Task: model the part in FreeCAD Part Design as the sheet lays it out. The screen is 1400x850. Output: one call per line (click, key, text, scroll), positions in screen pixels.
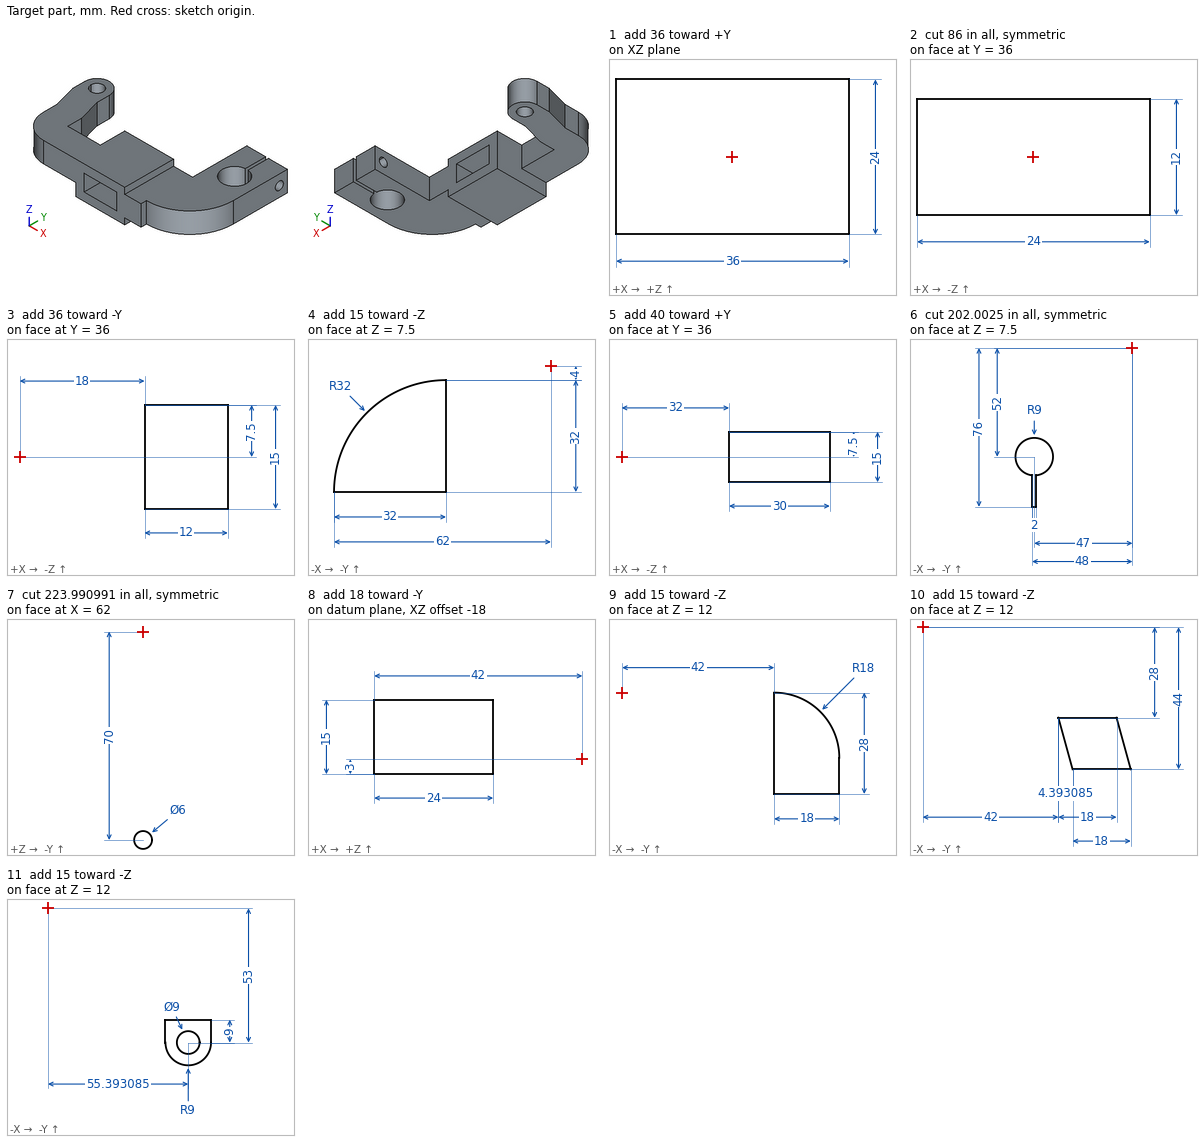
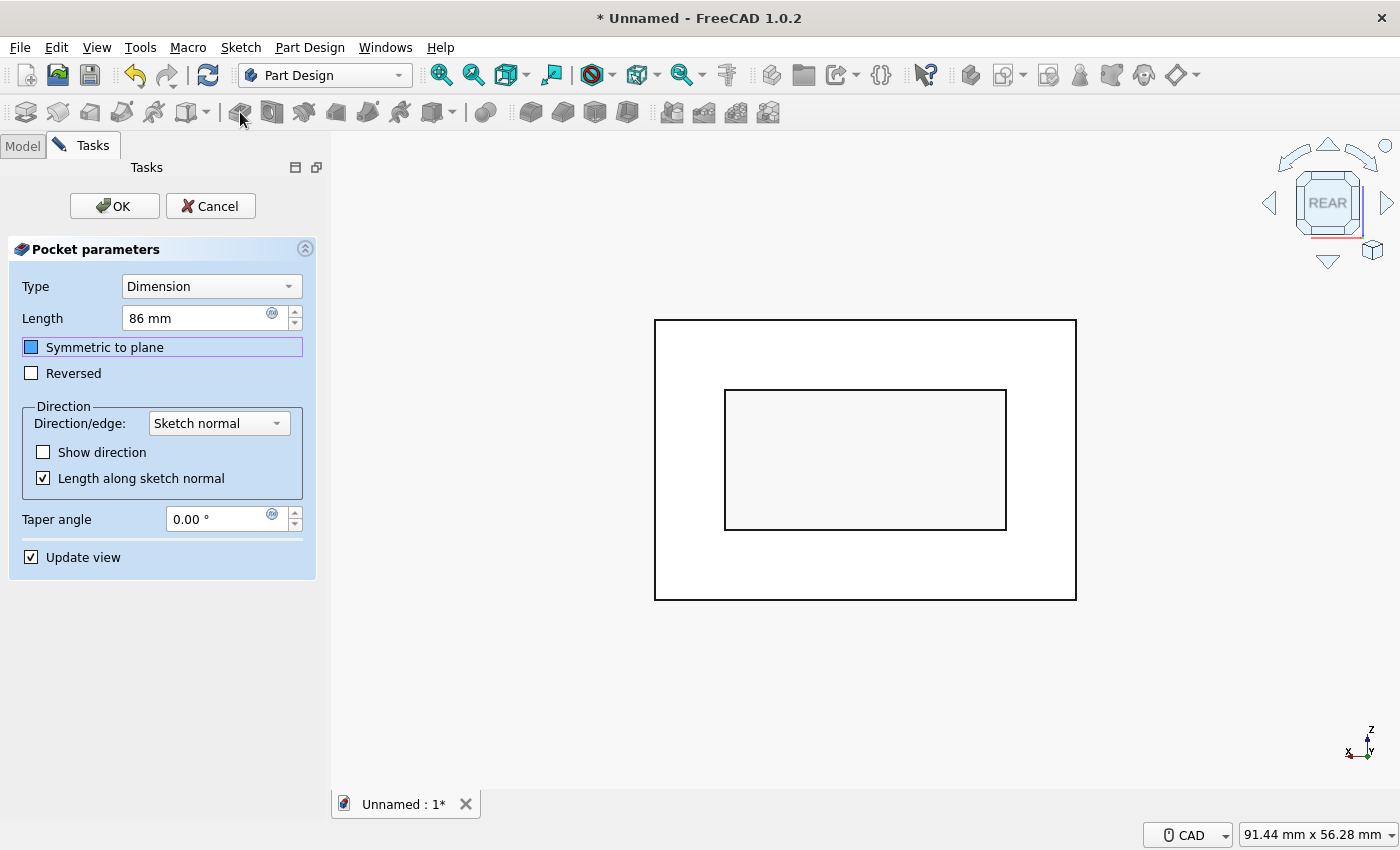
click(30, 347)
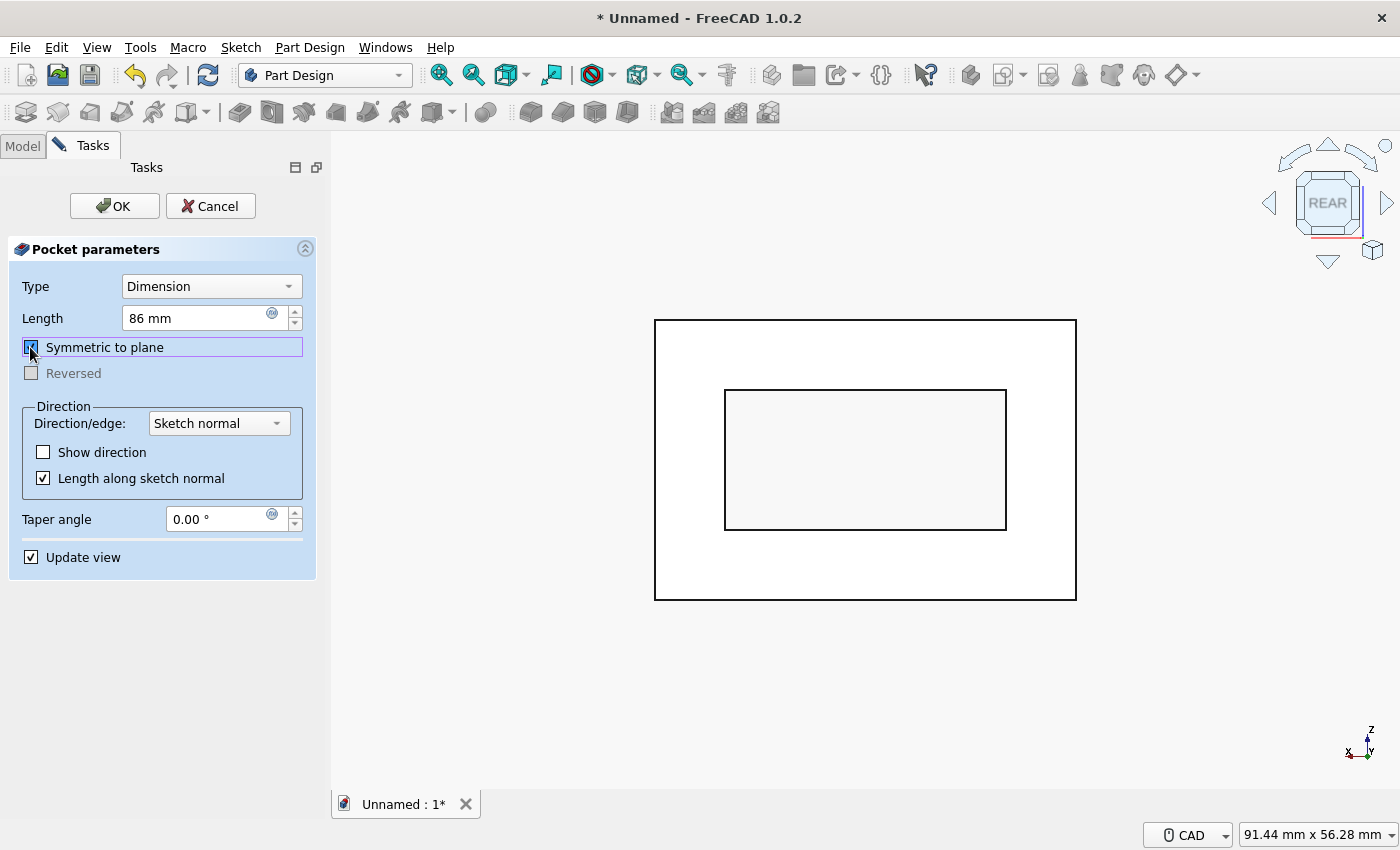
click(115, 206)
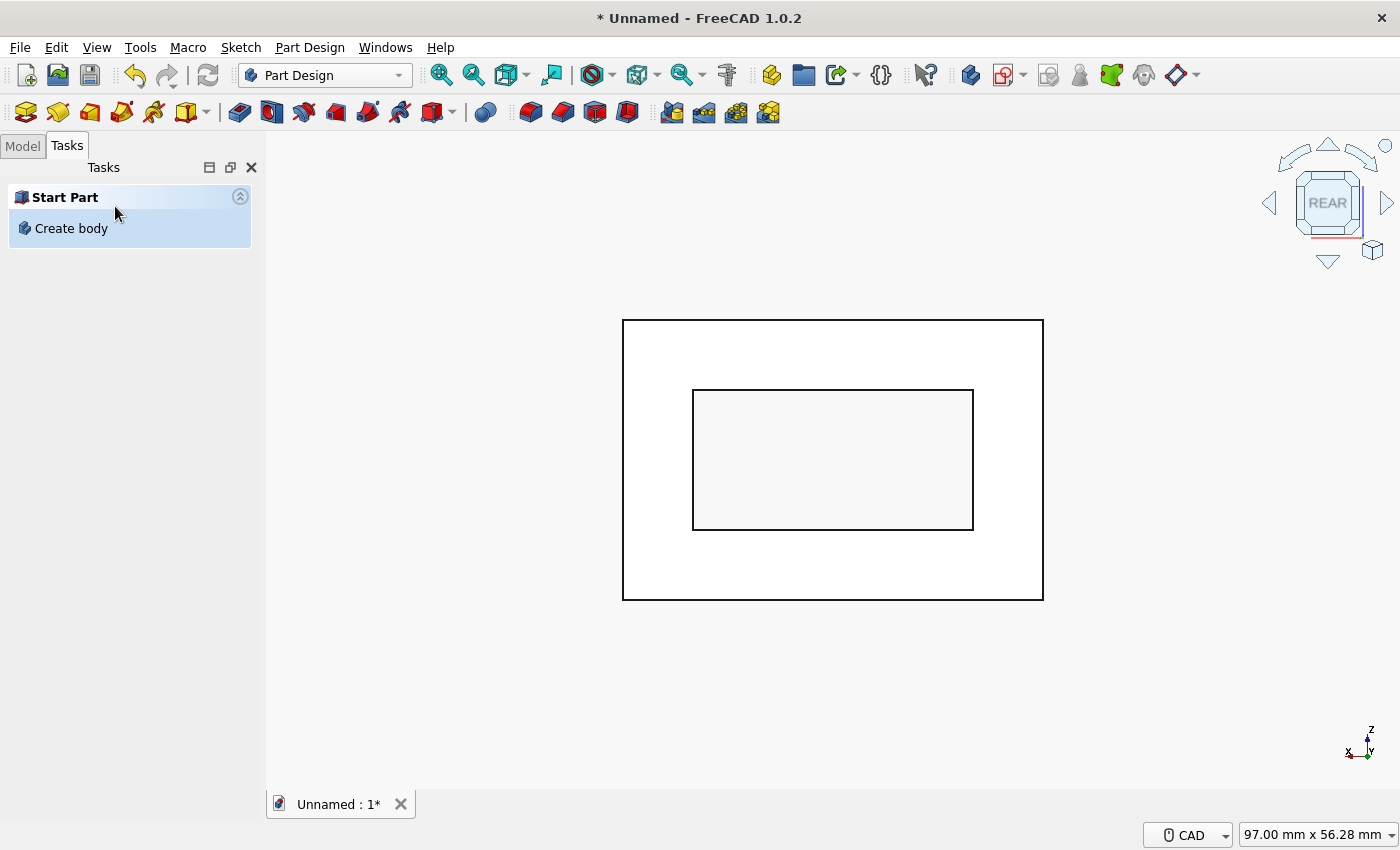
click(442, 76)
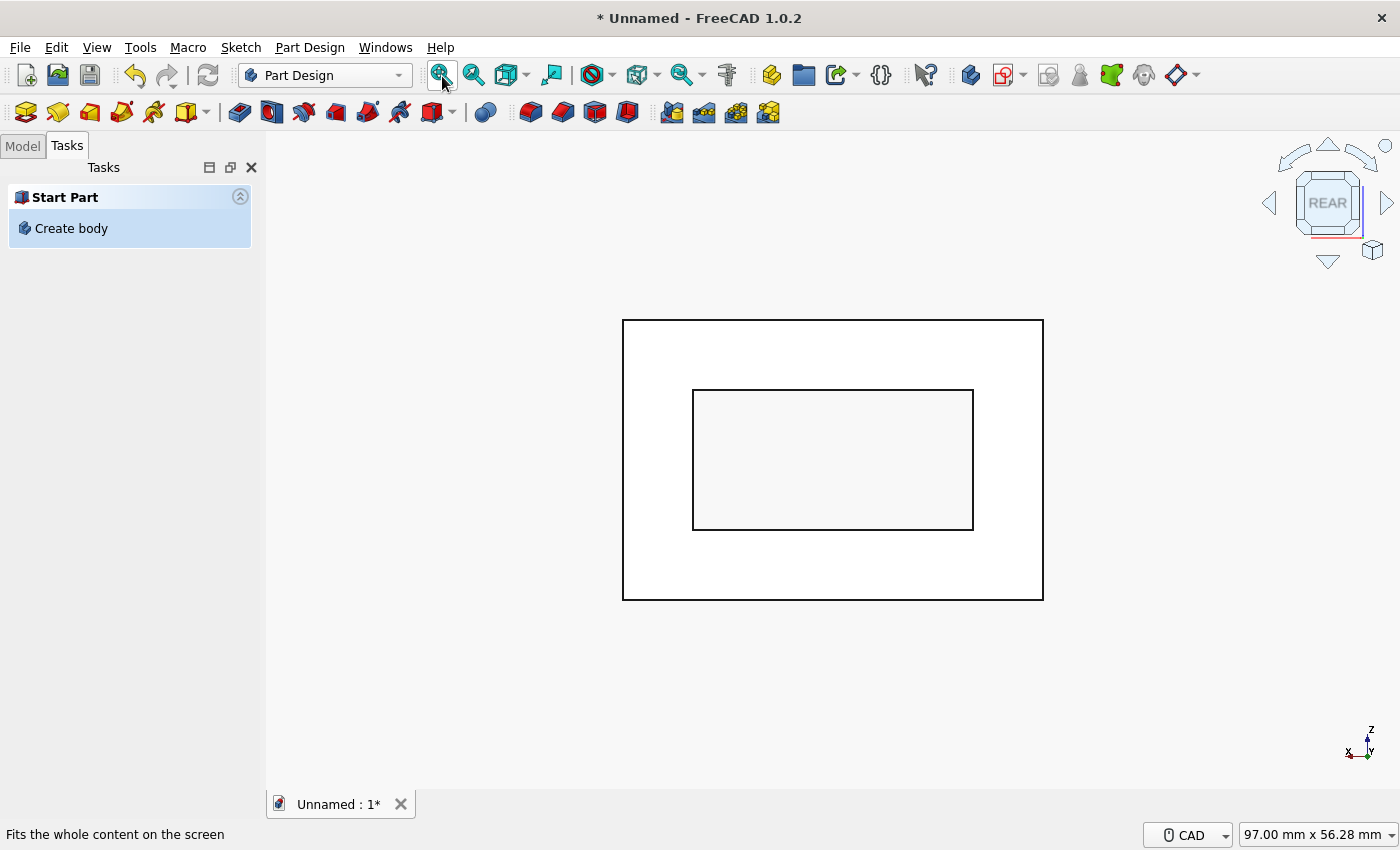
click(1013, 379)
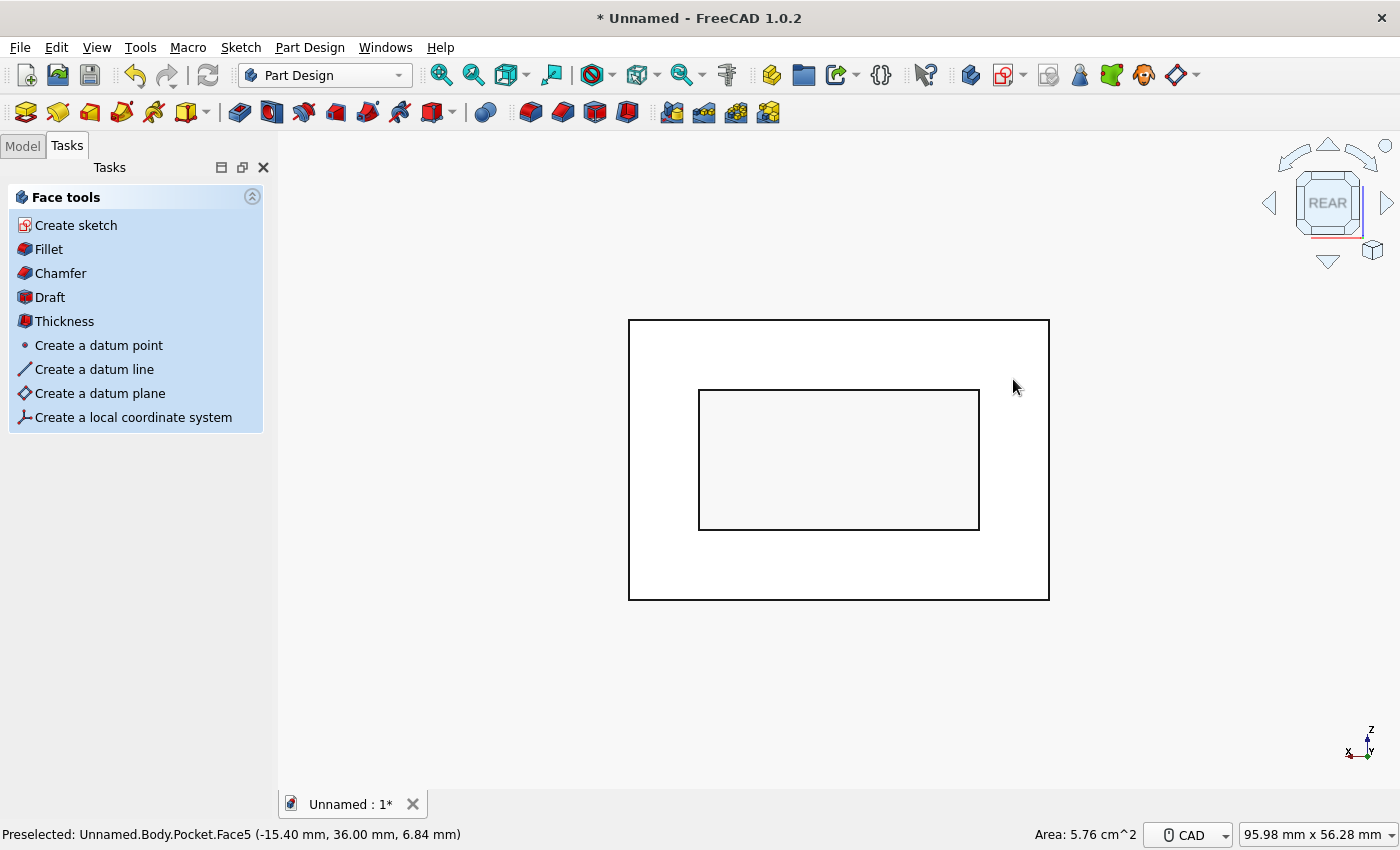
click(1004, 76)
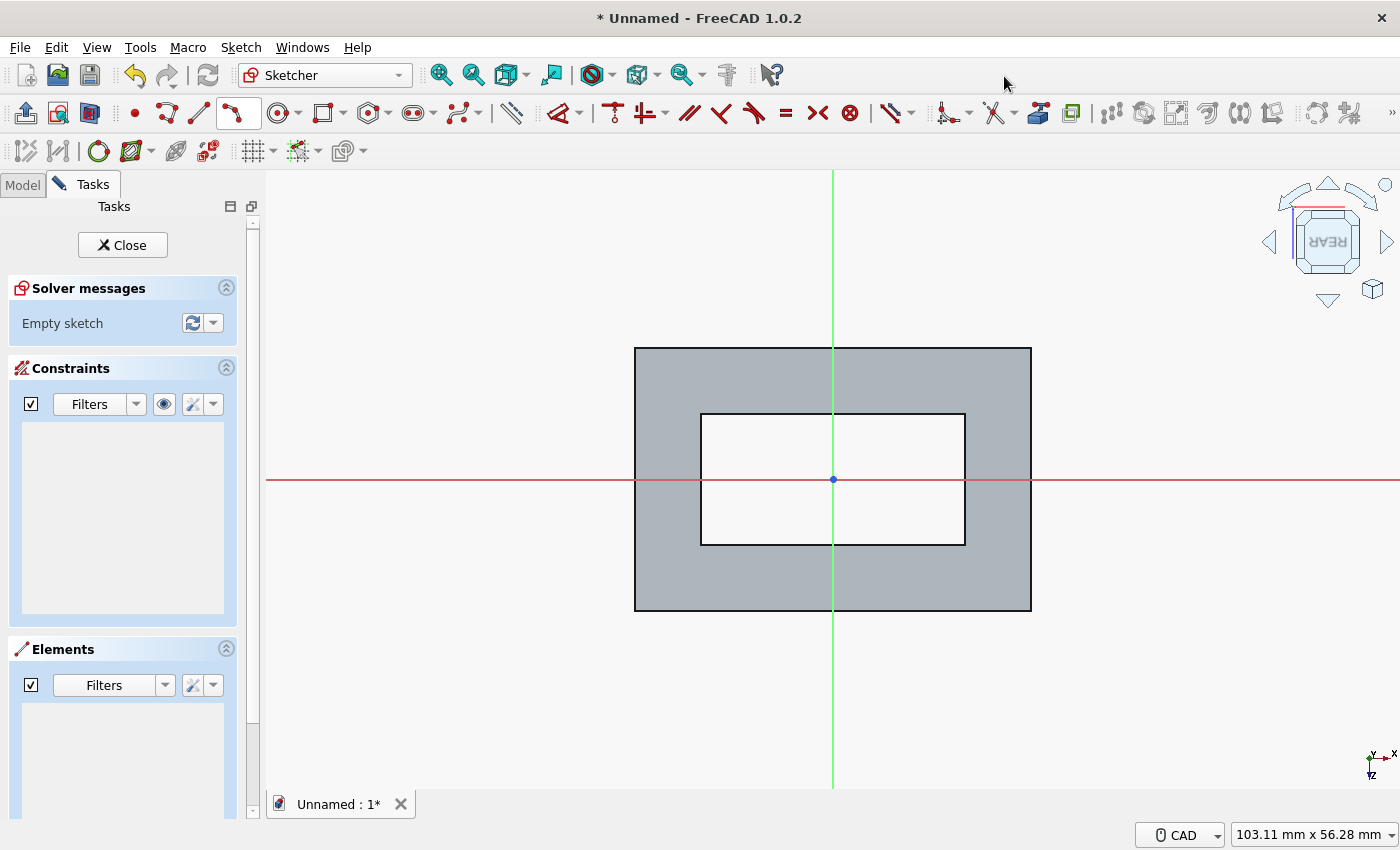
scroll(1235, 479, up, 3)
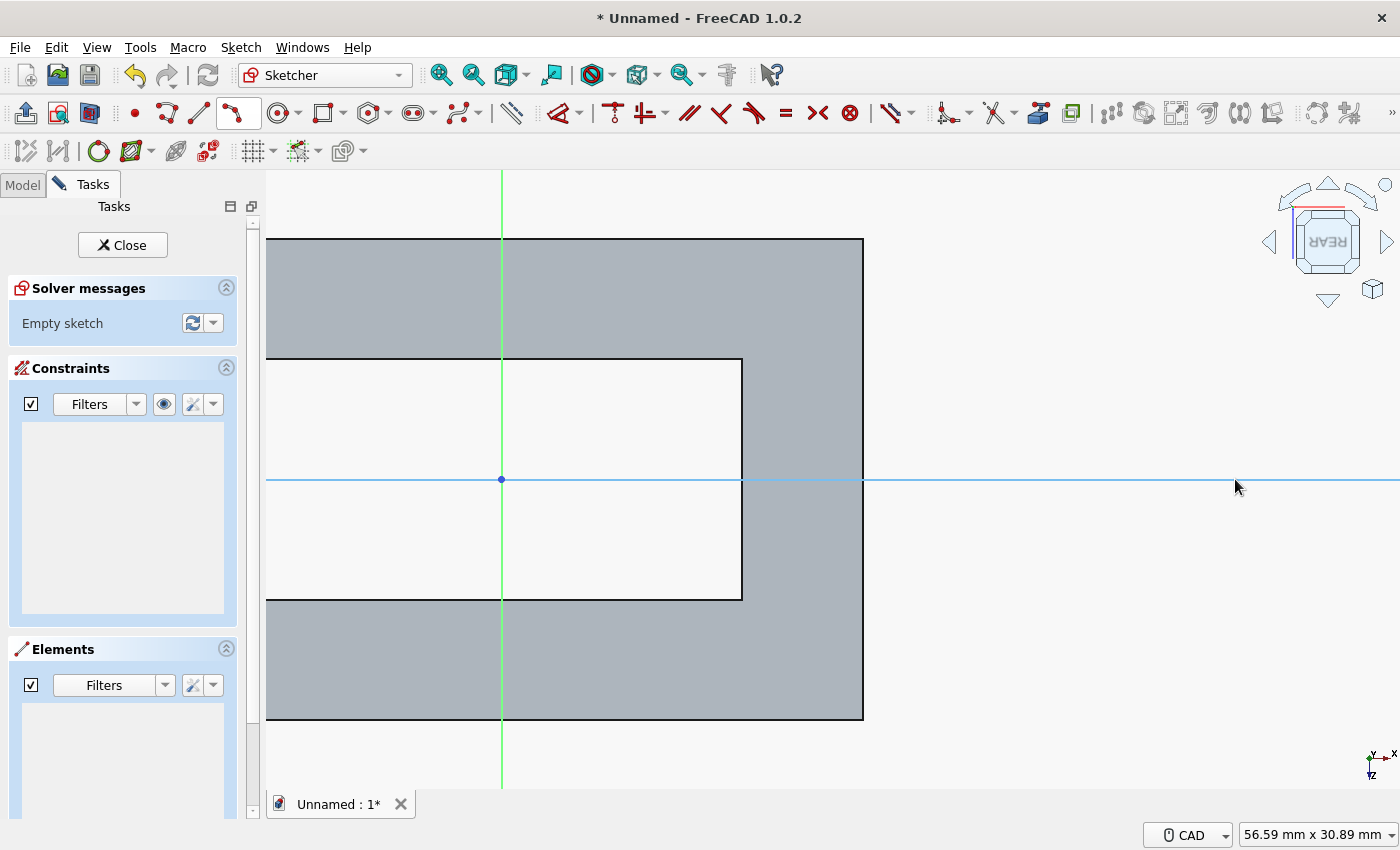
key(g)
key(r)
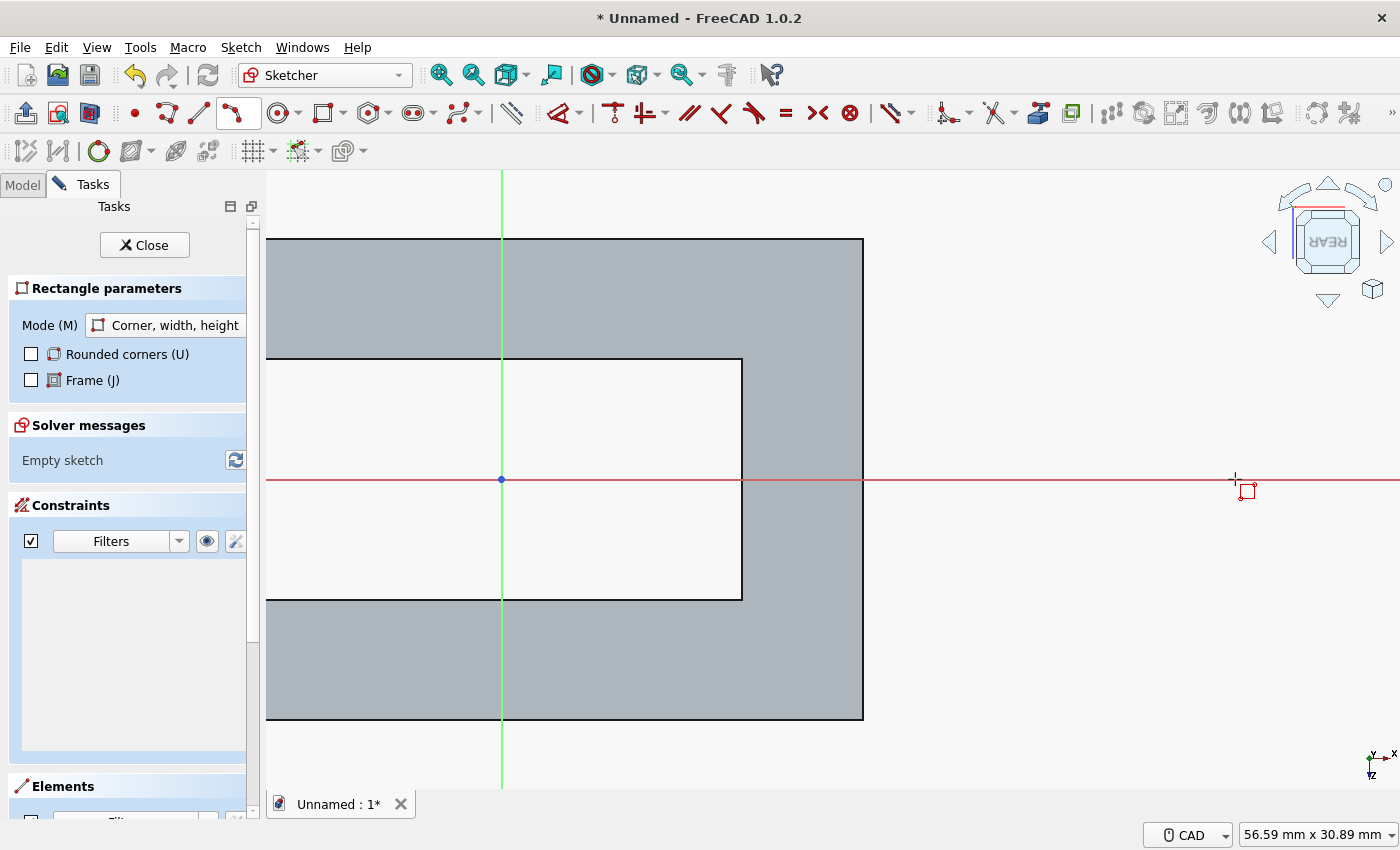
click(863, 329)
click(1103, 630)
key(Escape)